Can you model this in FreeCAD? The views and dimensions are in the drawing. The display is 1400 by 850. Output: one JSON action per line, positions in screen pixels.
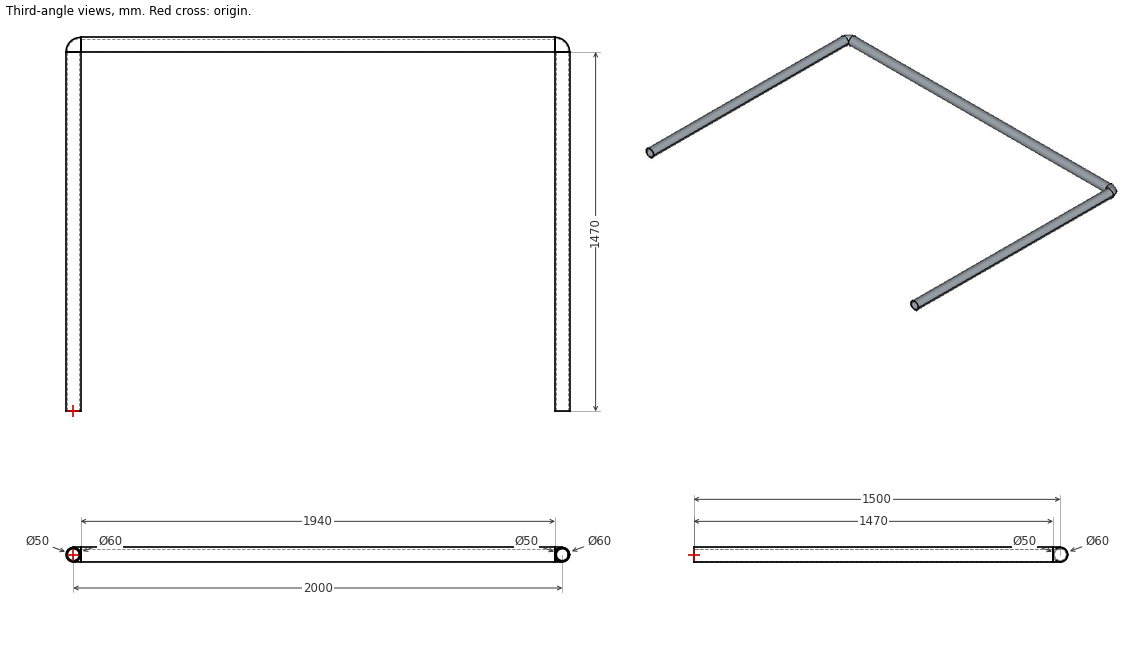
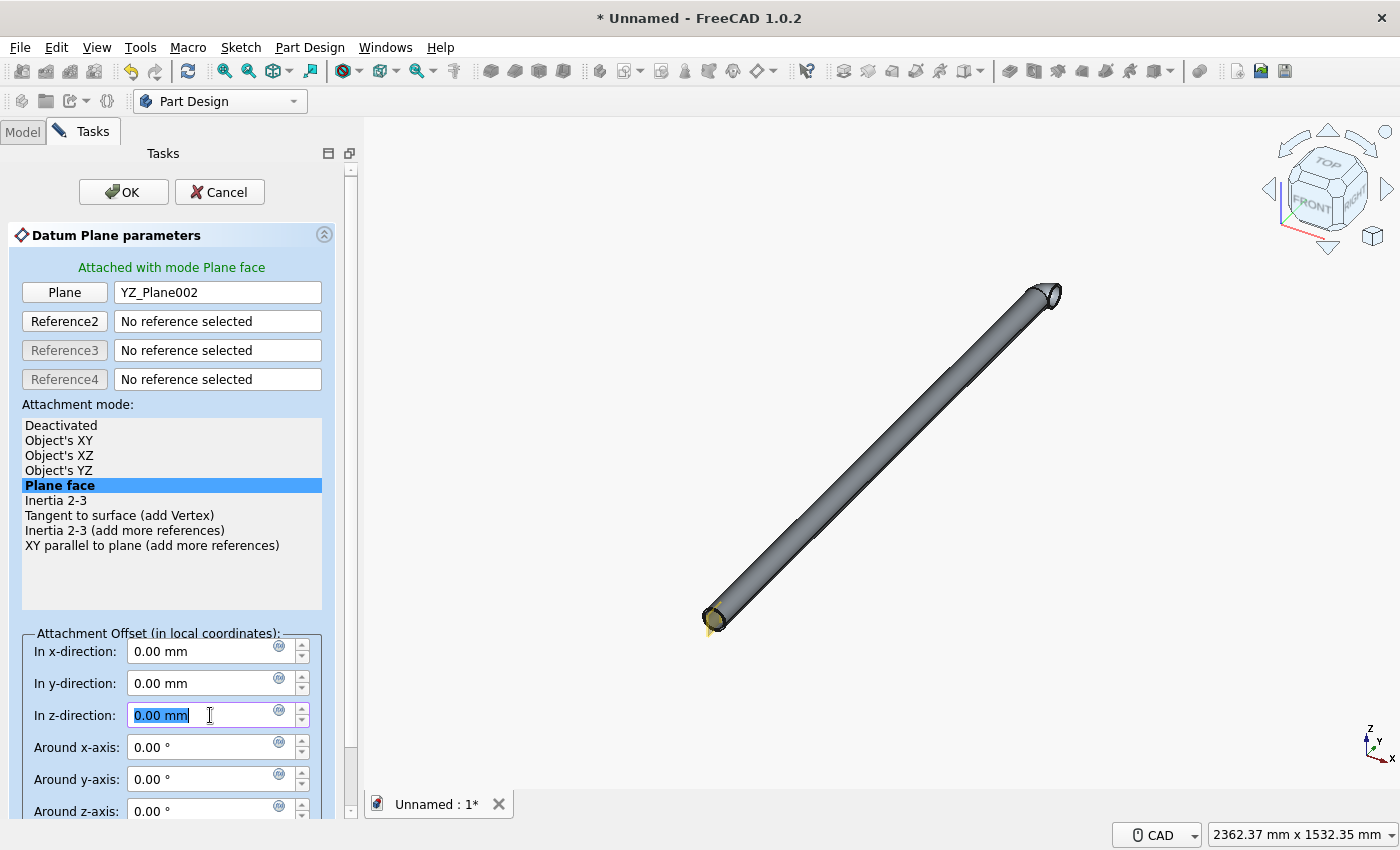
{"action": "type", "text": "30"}
{"action": "key", "text": "Tab"}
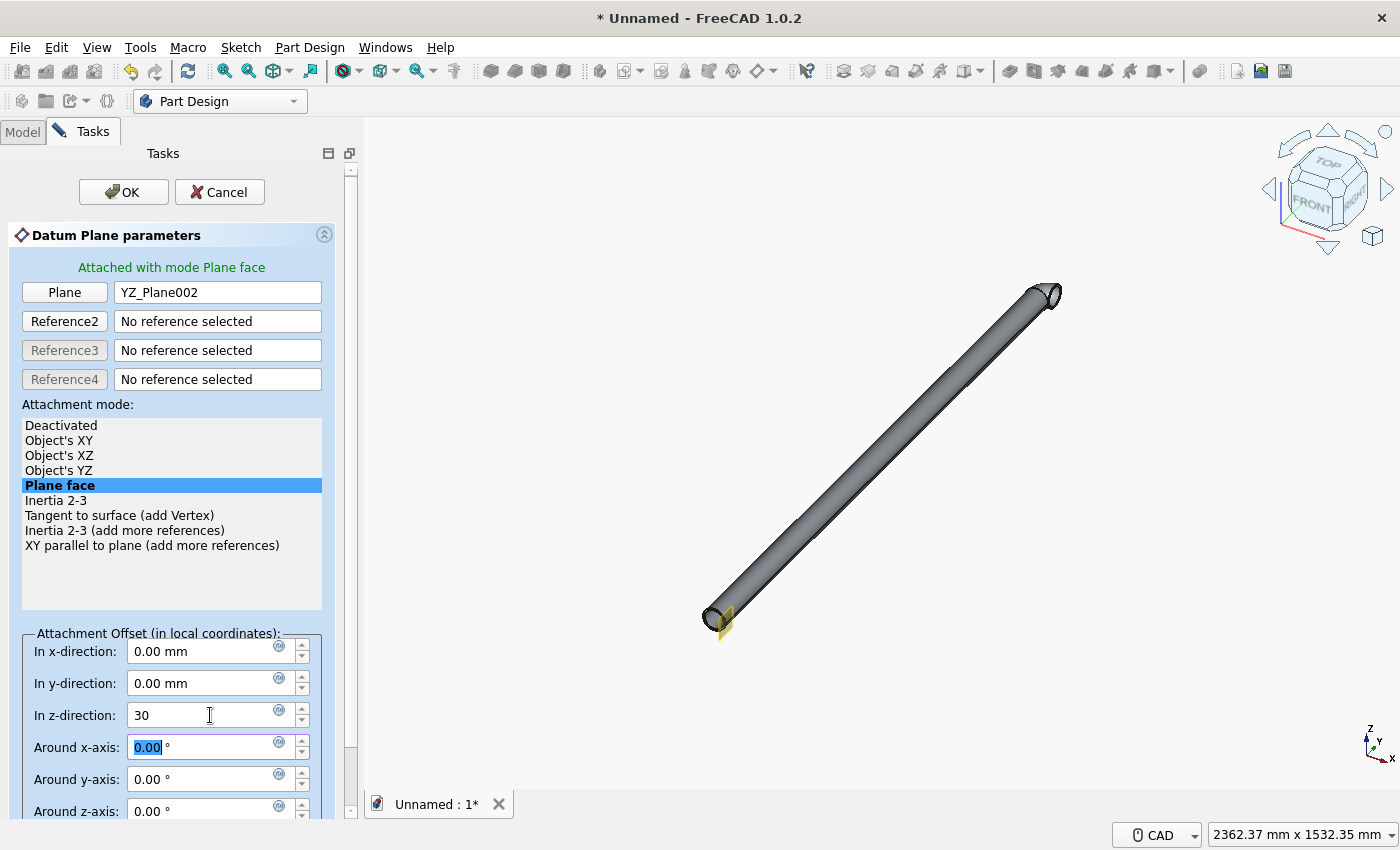
{"action": "left_click", "coordinate": [124, 192]}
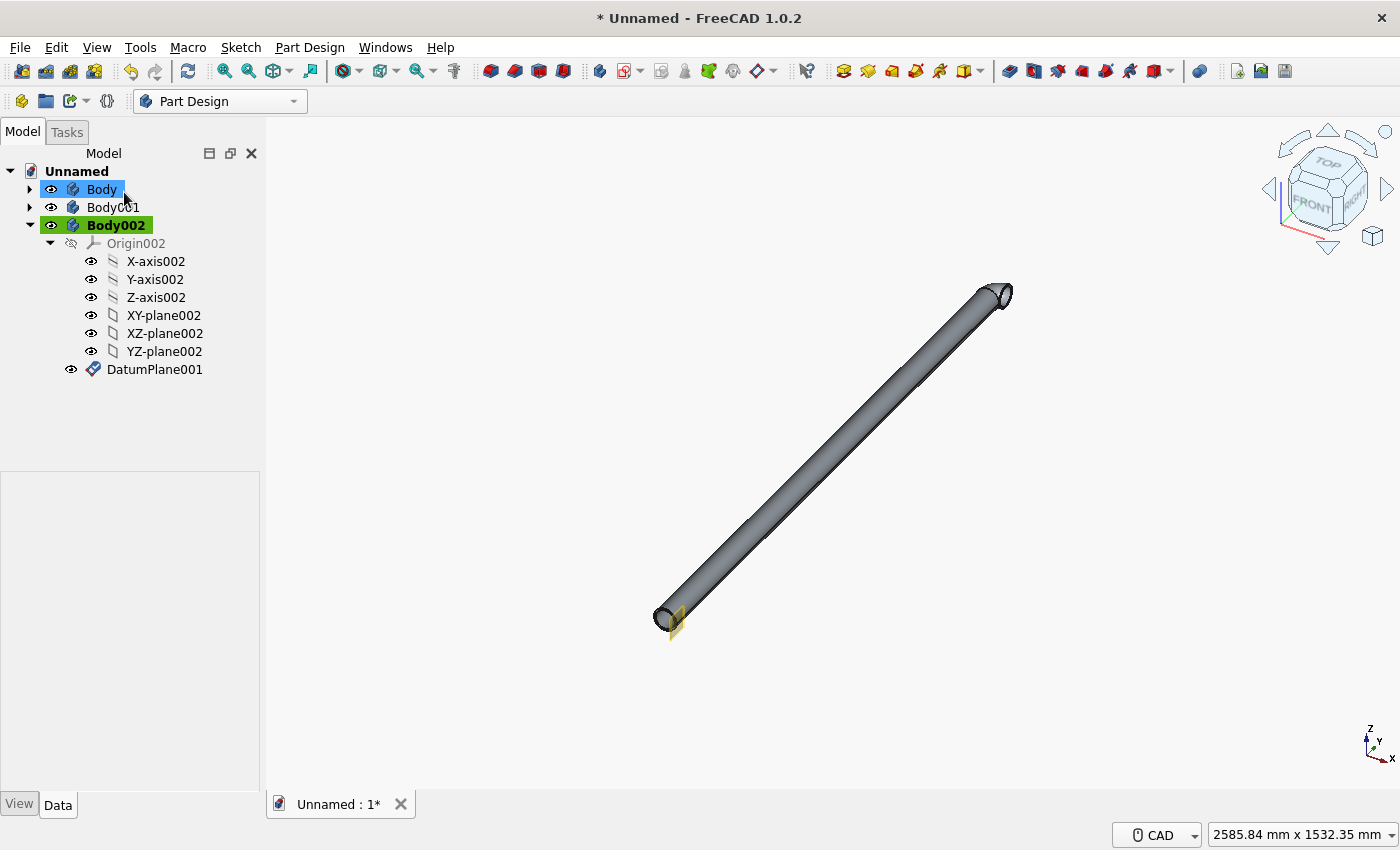
{"action": "left_click", "coordinate": [116, 369]}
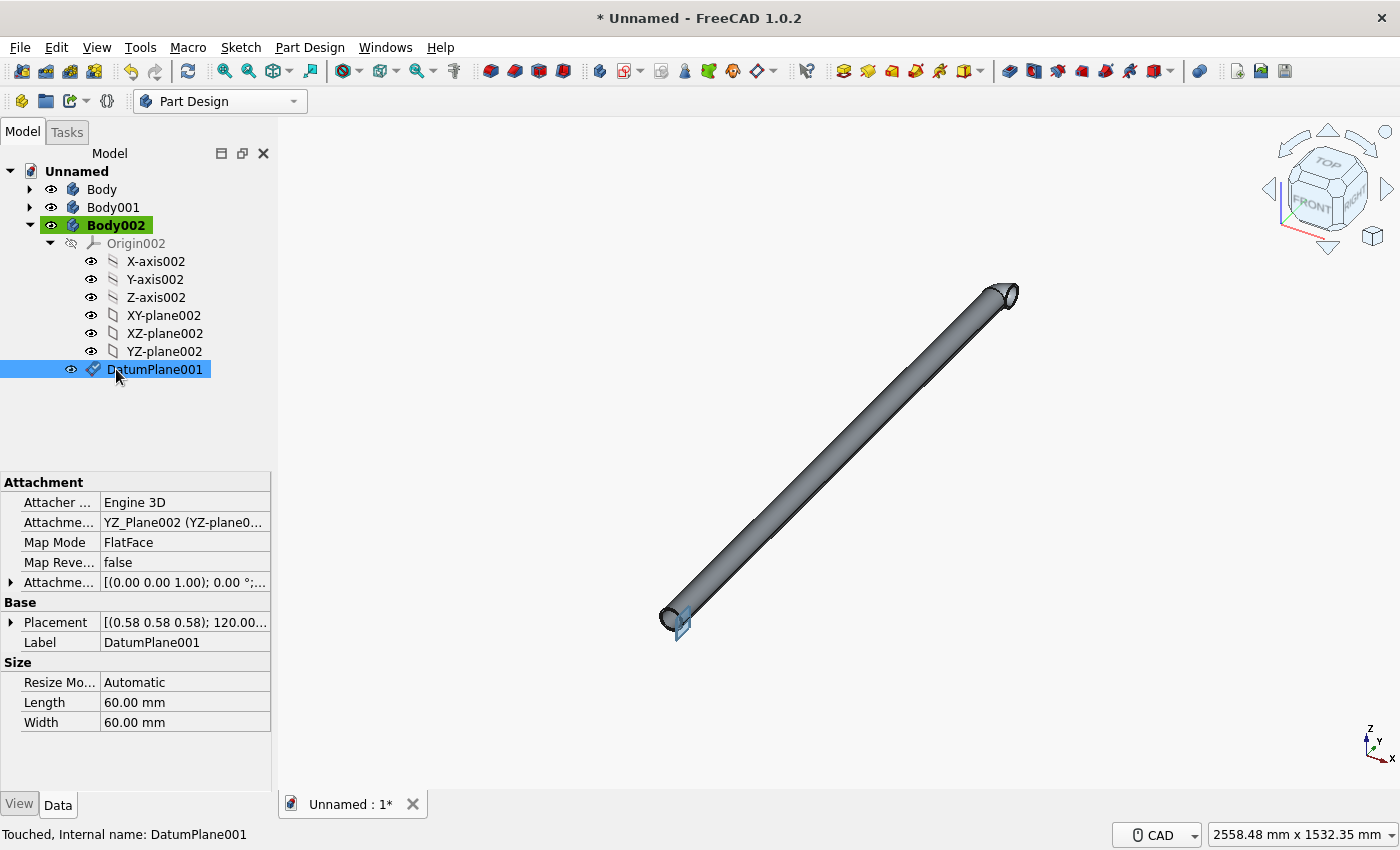
{"action": "left_click", "coordinate": [624, 72]}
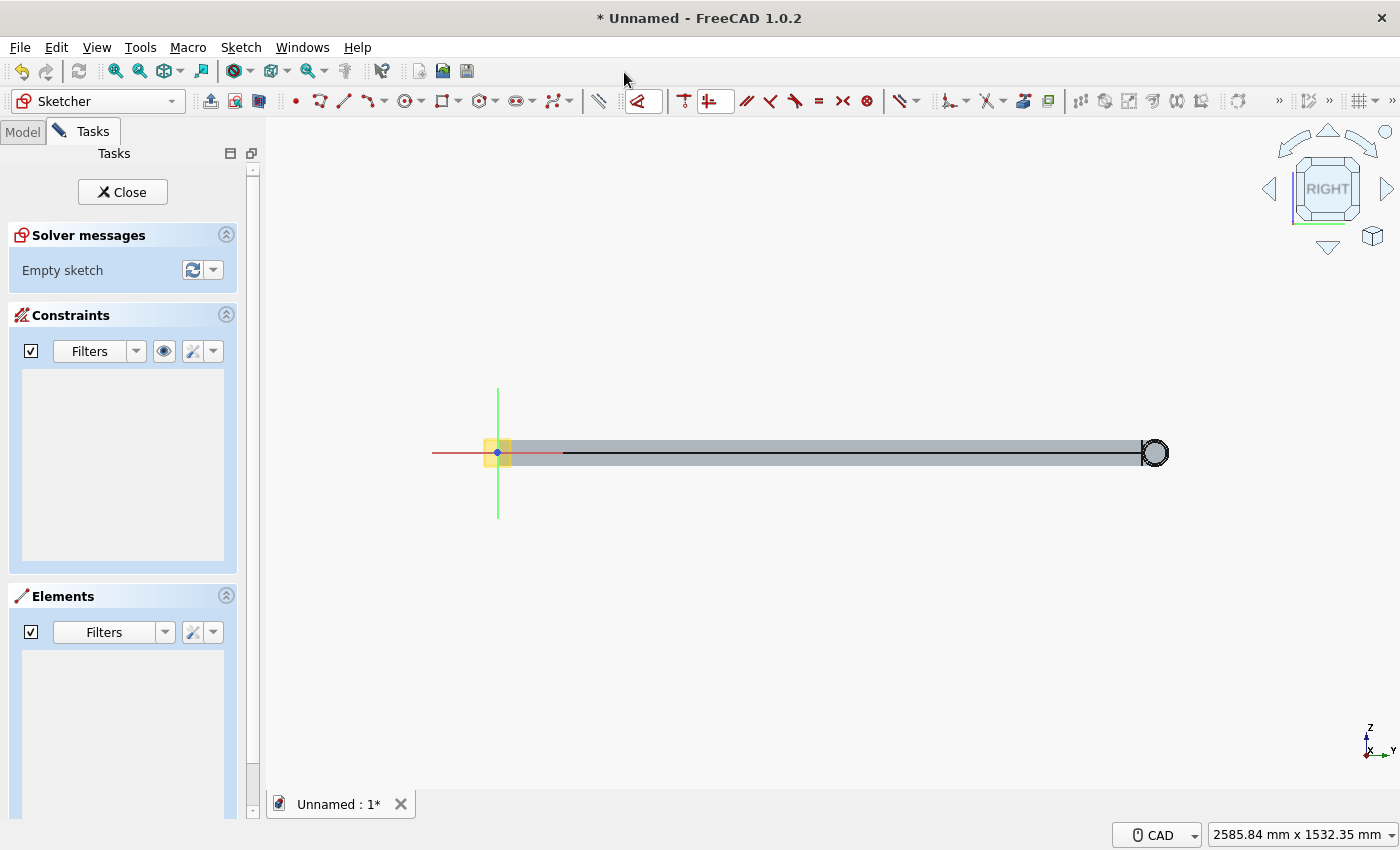
{"action": "scroll", "coordinate": [1181, 453], "scroll_direction": "up", "scroll_amount": 14}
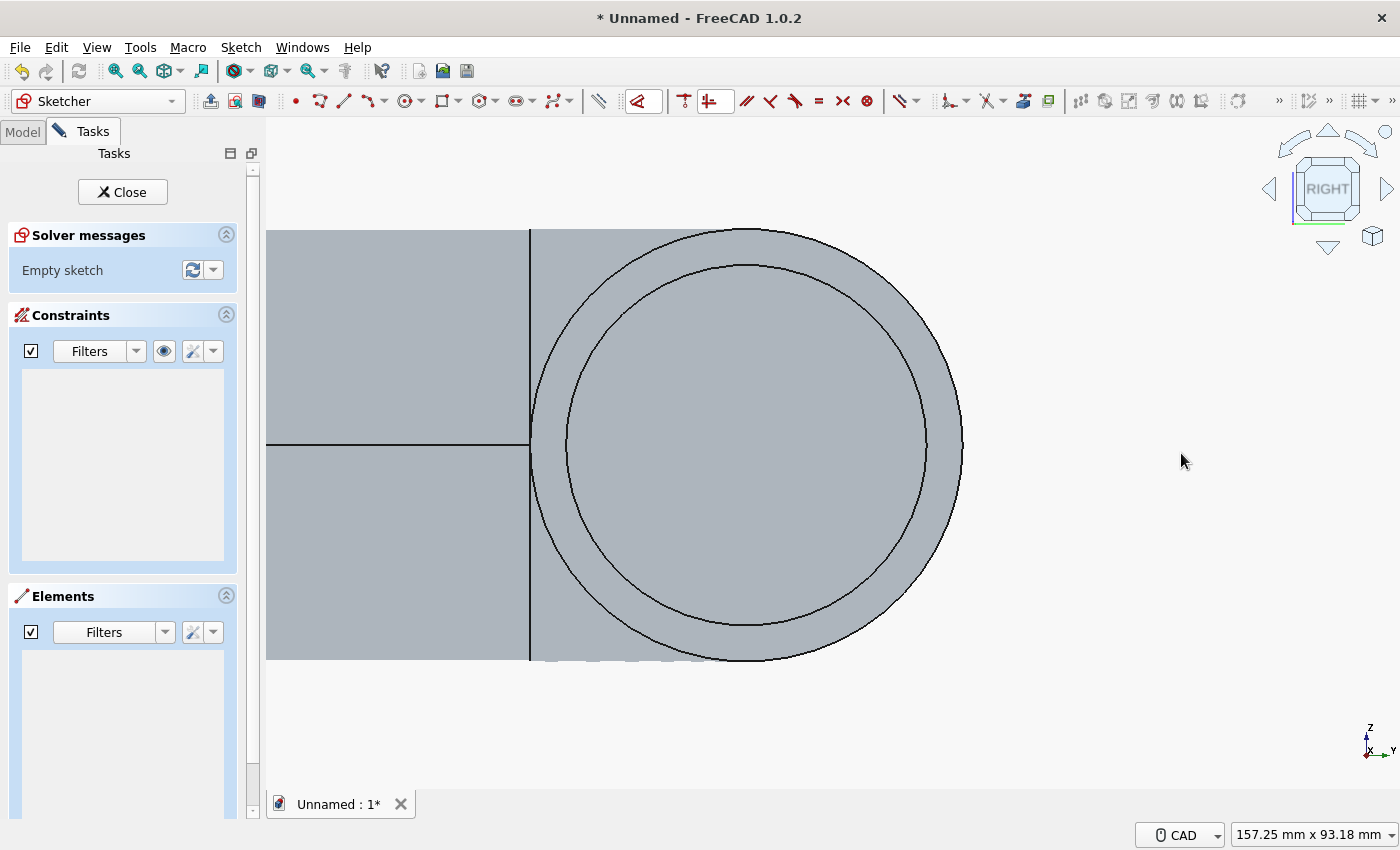
{"action": "left_click", "coordinate": [406, 102]}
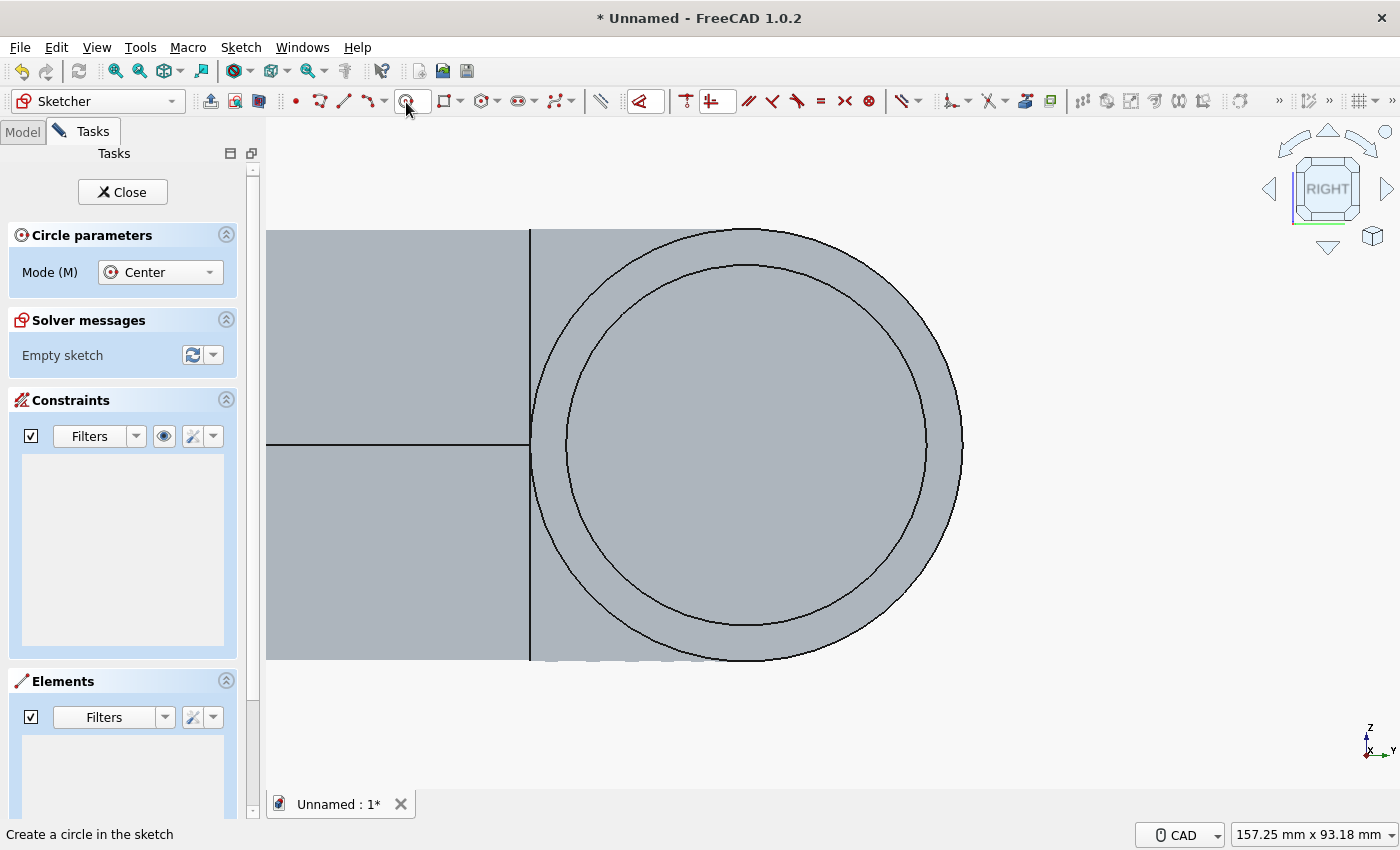
{"action": "left_click", "coordinate": [746, 445]}
{"action": "mouse_move", "coordinate": [899, 292]}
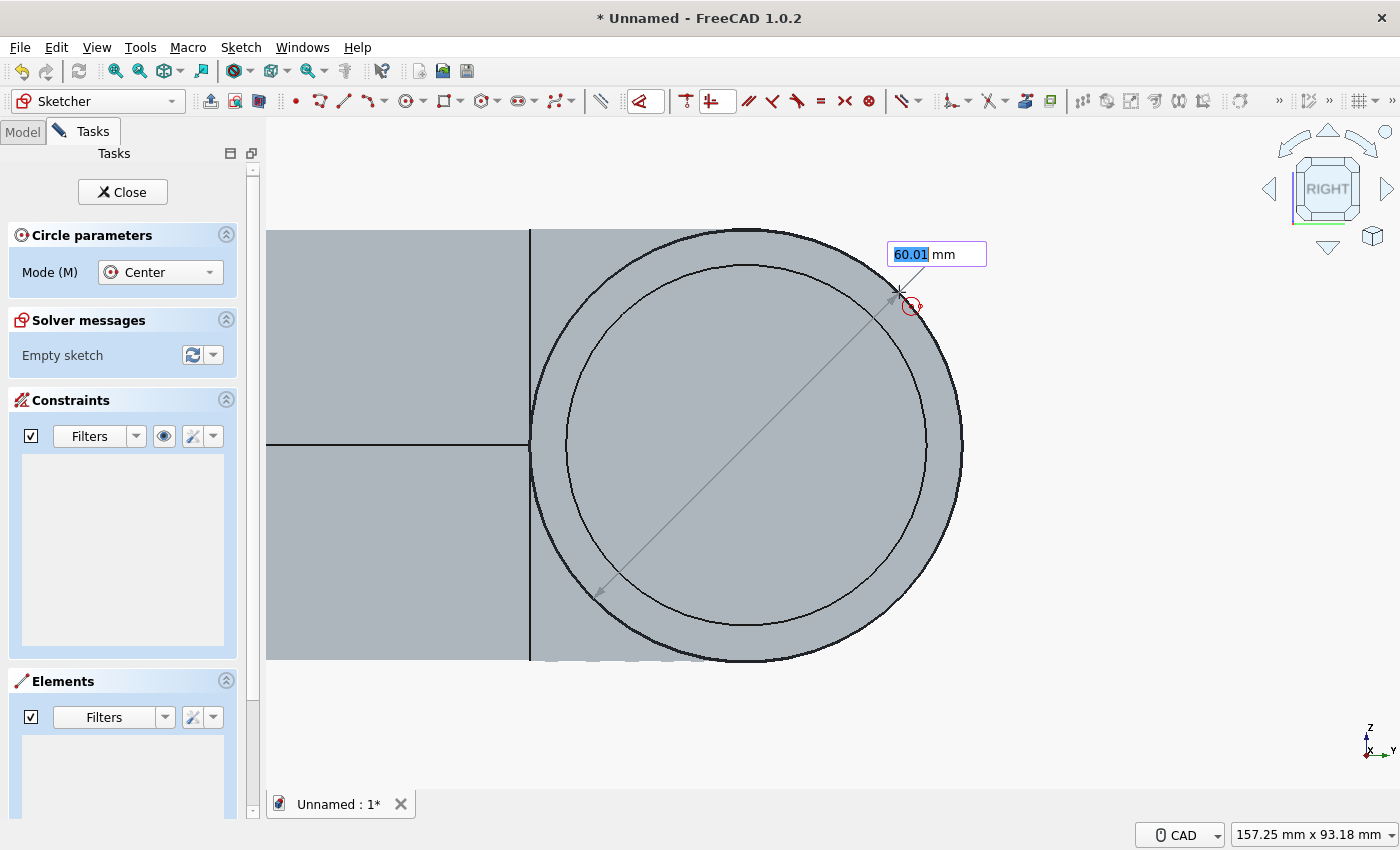
{"action": "type", "text": "60"}
{"action": "key", "text": "Return"}